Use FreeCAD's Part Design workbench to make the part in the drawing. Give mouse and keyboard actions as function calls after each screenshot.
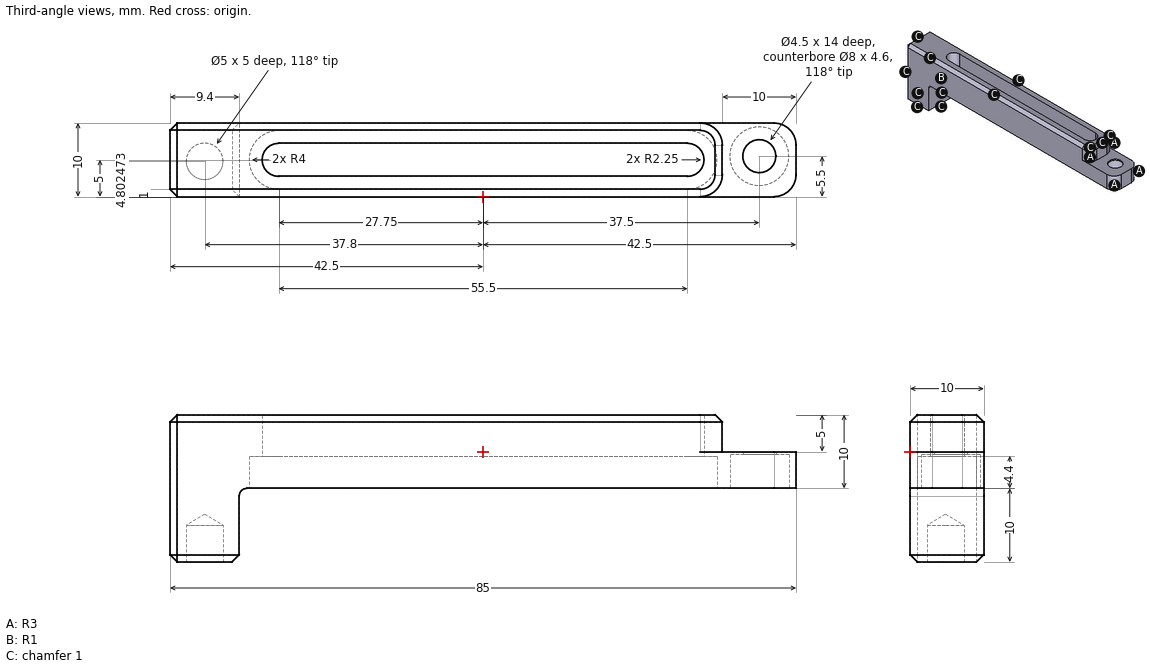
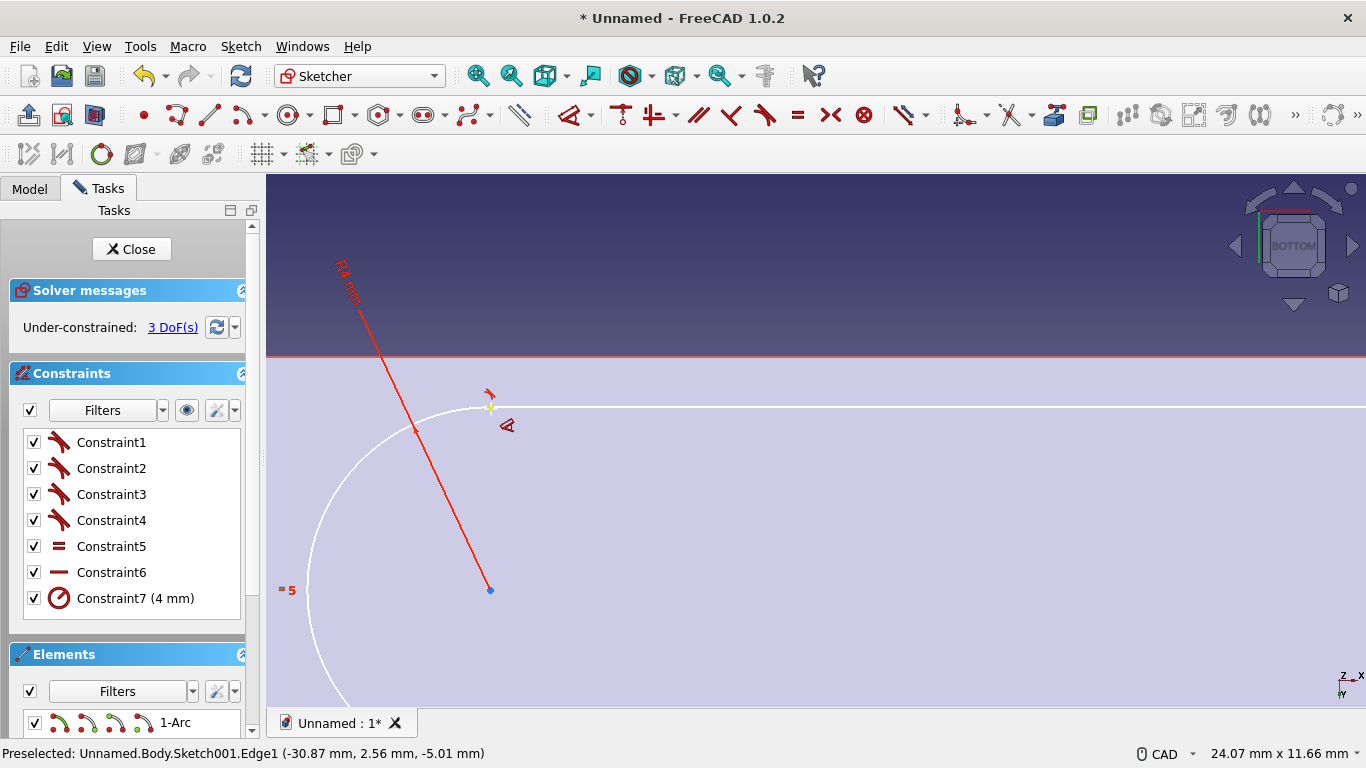
click(490, 407)
click(456, 382)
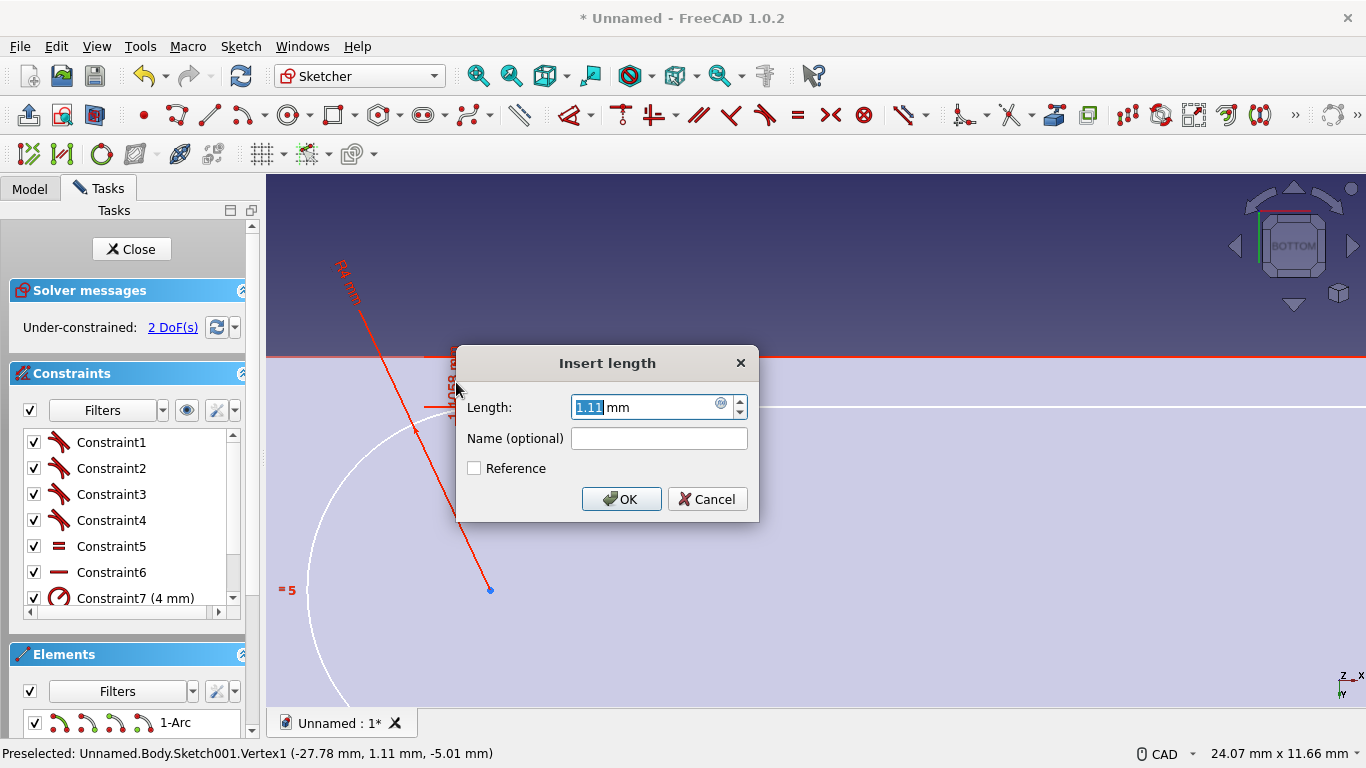
text(1)
key(Return)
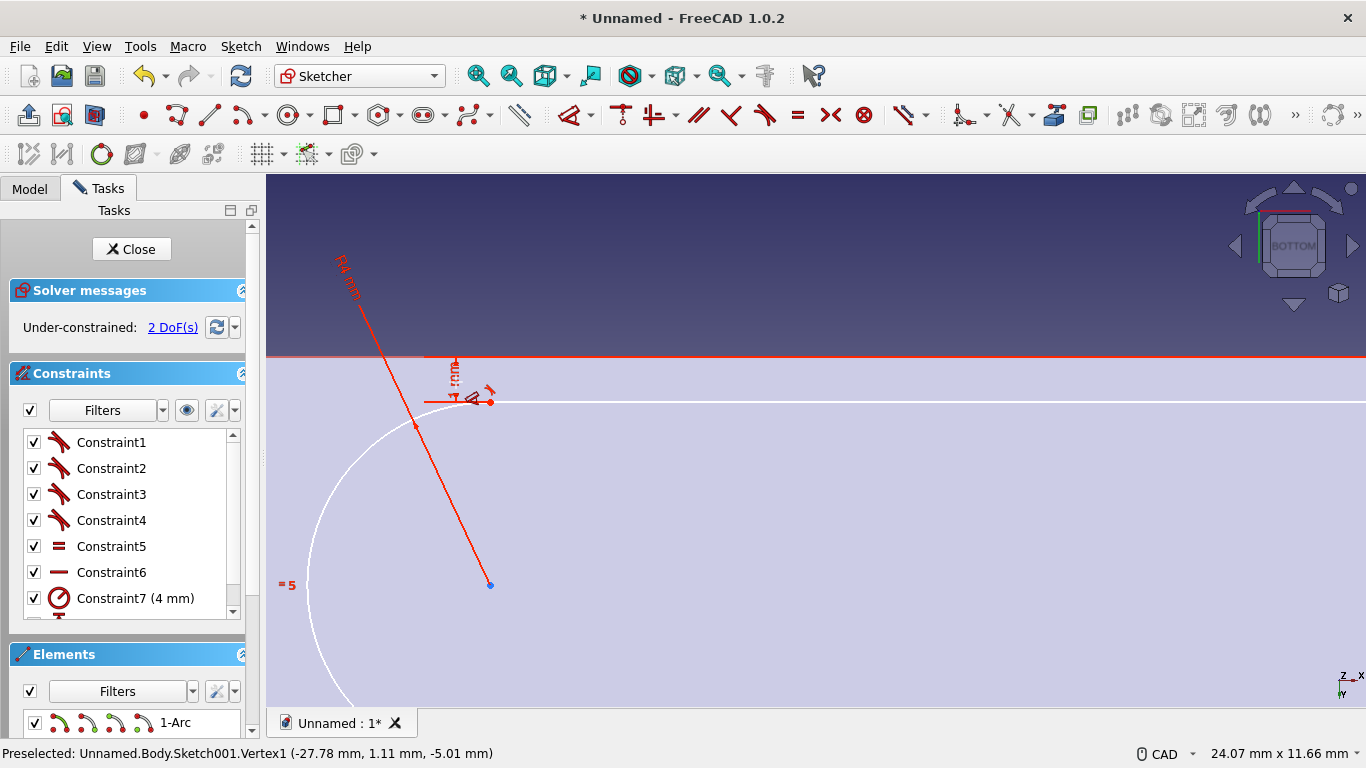
scroll(491, 410, down, 8)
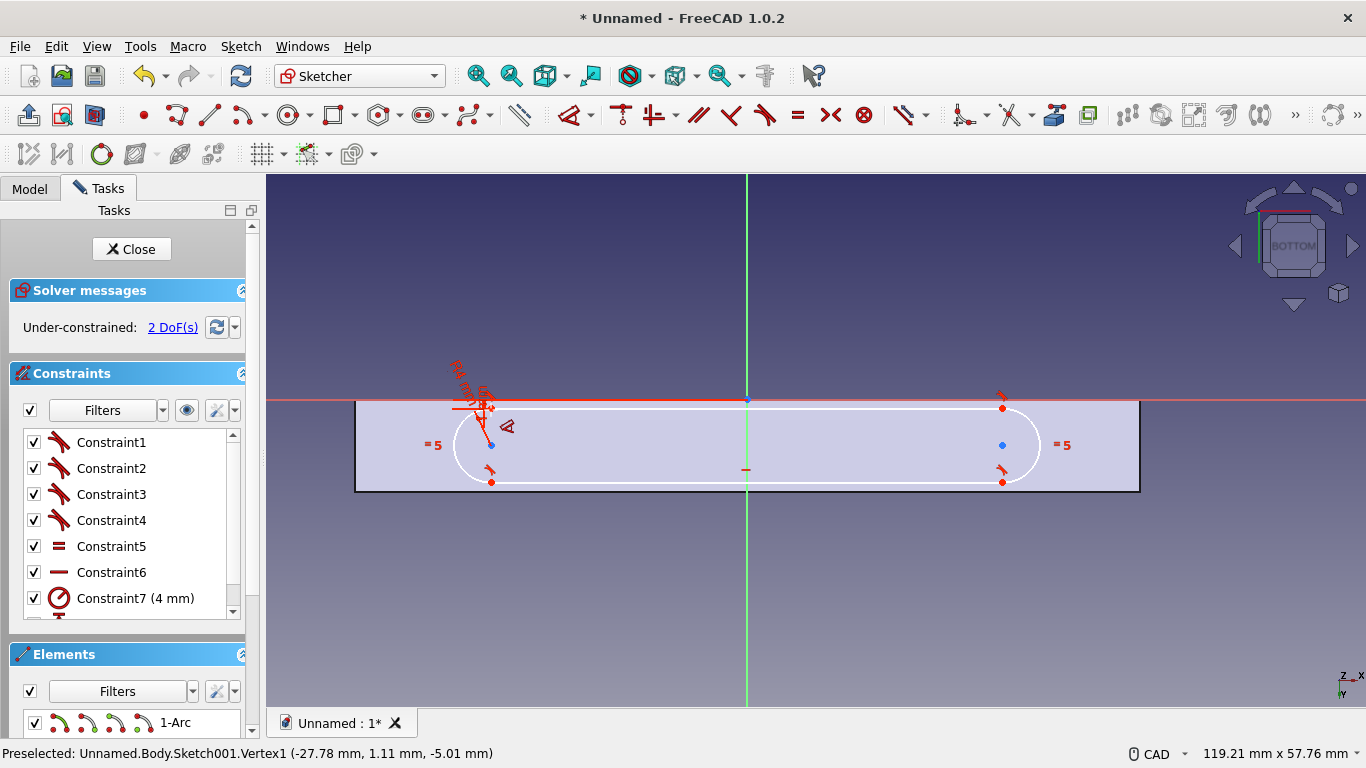
scroll(593, 409, up, 3)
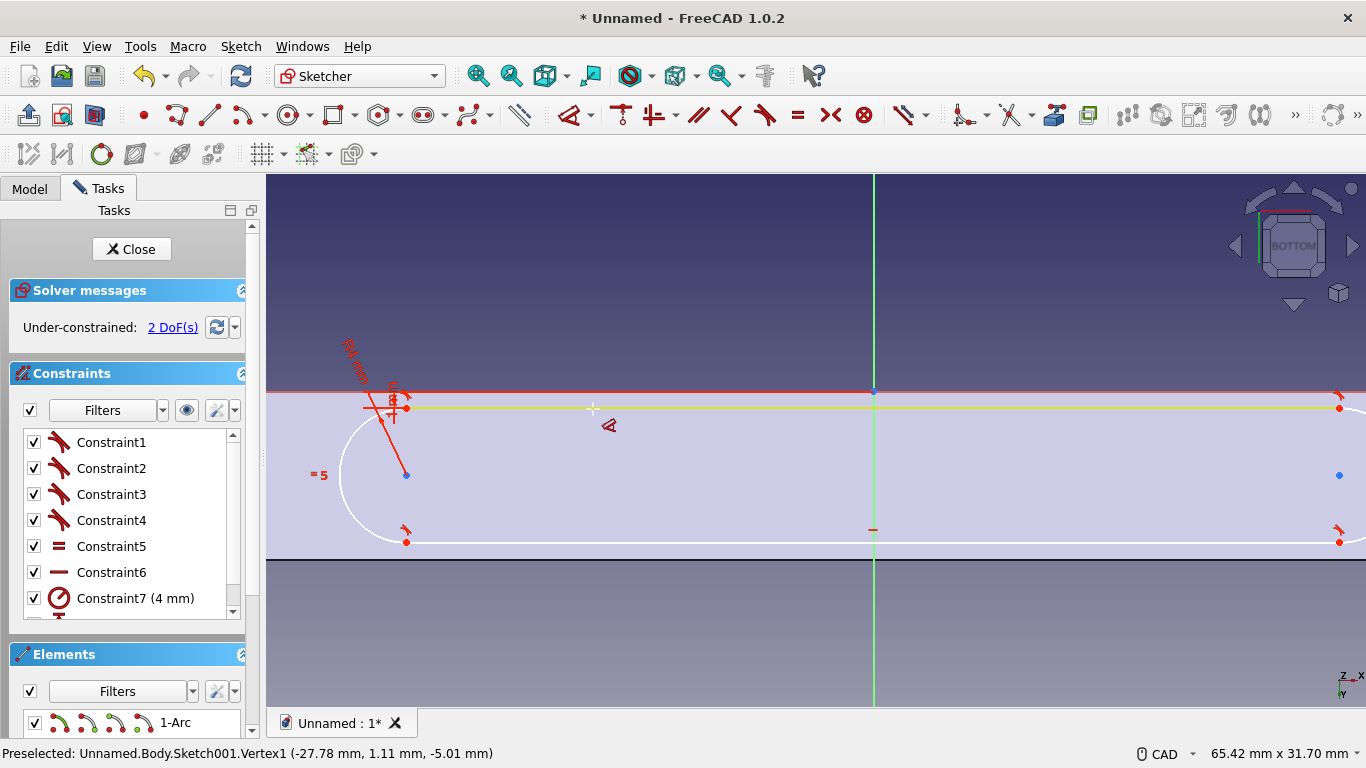
click(593, 408)
click(804, 374)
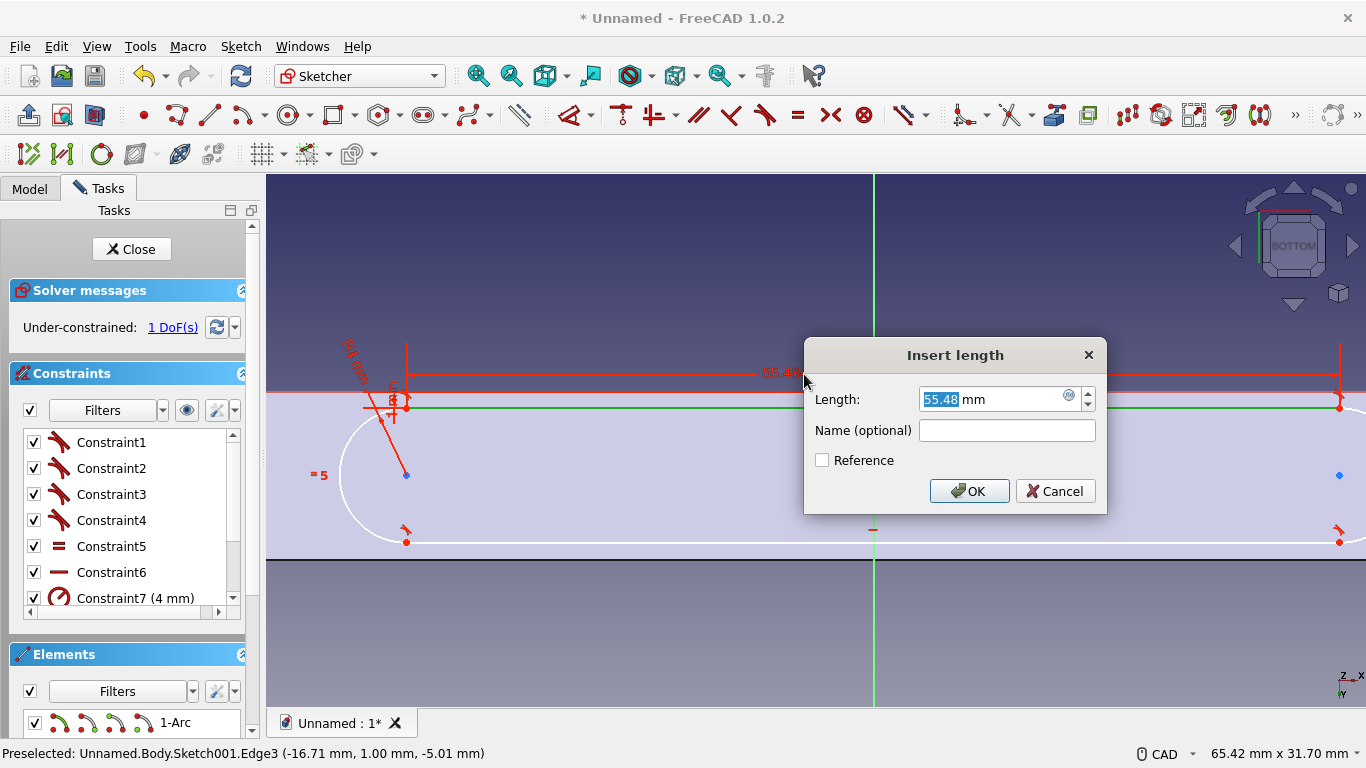
text(55.5)
key(Return)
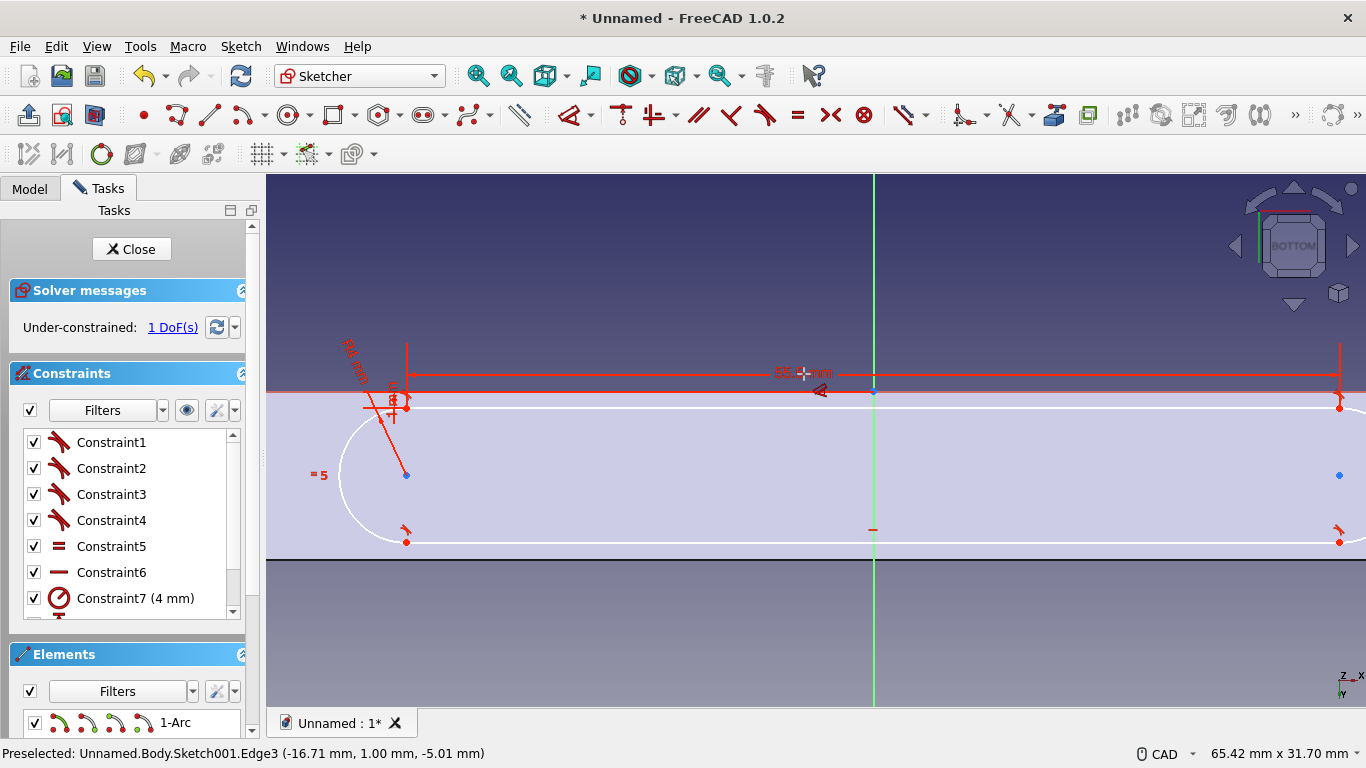
click(407, 408)
click(640, 358)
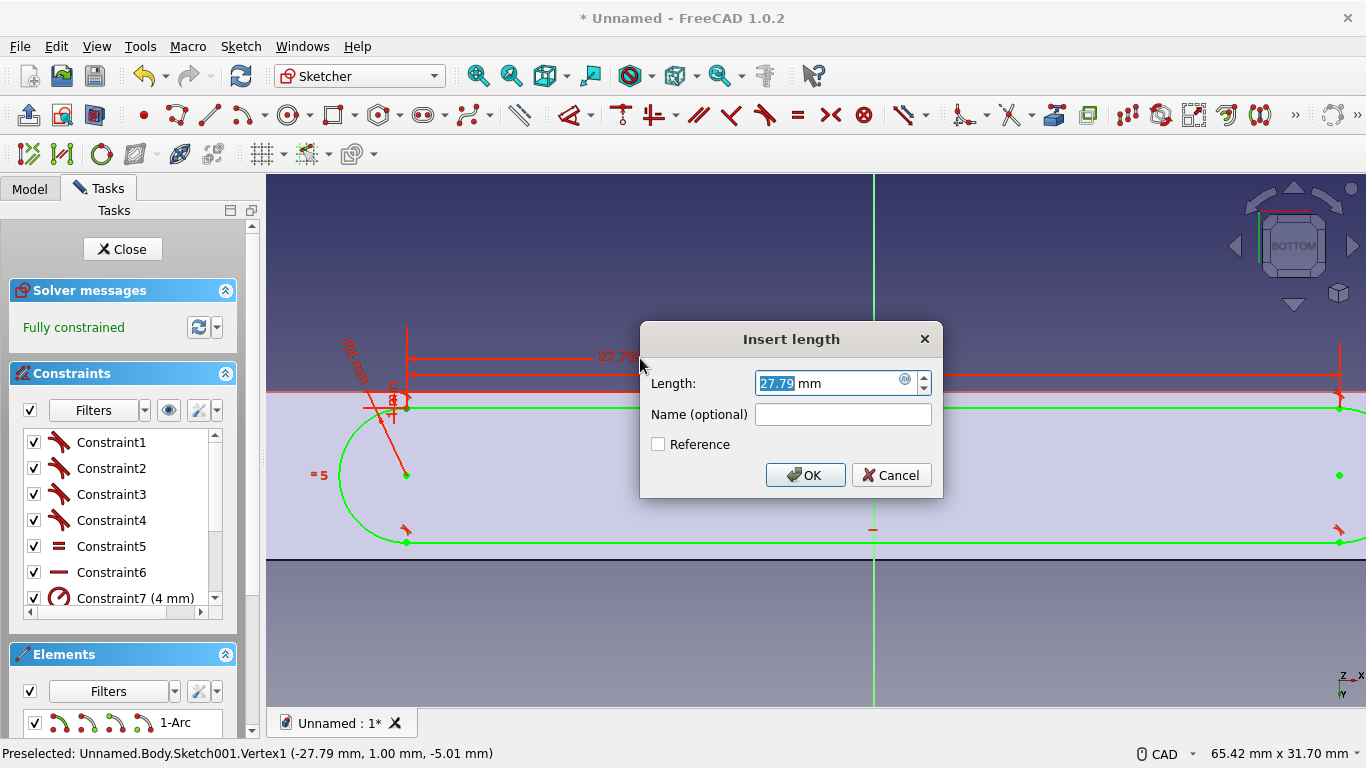
text(27.75)
key(Return)
key(Escape)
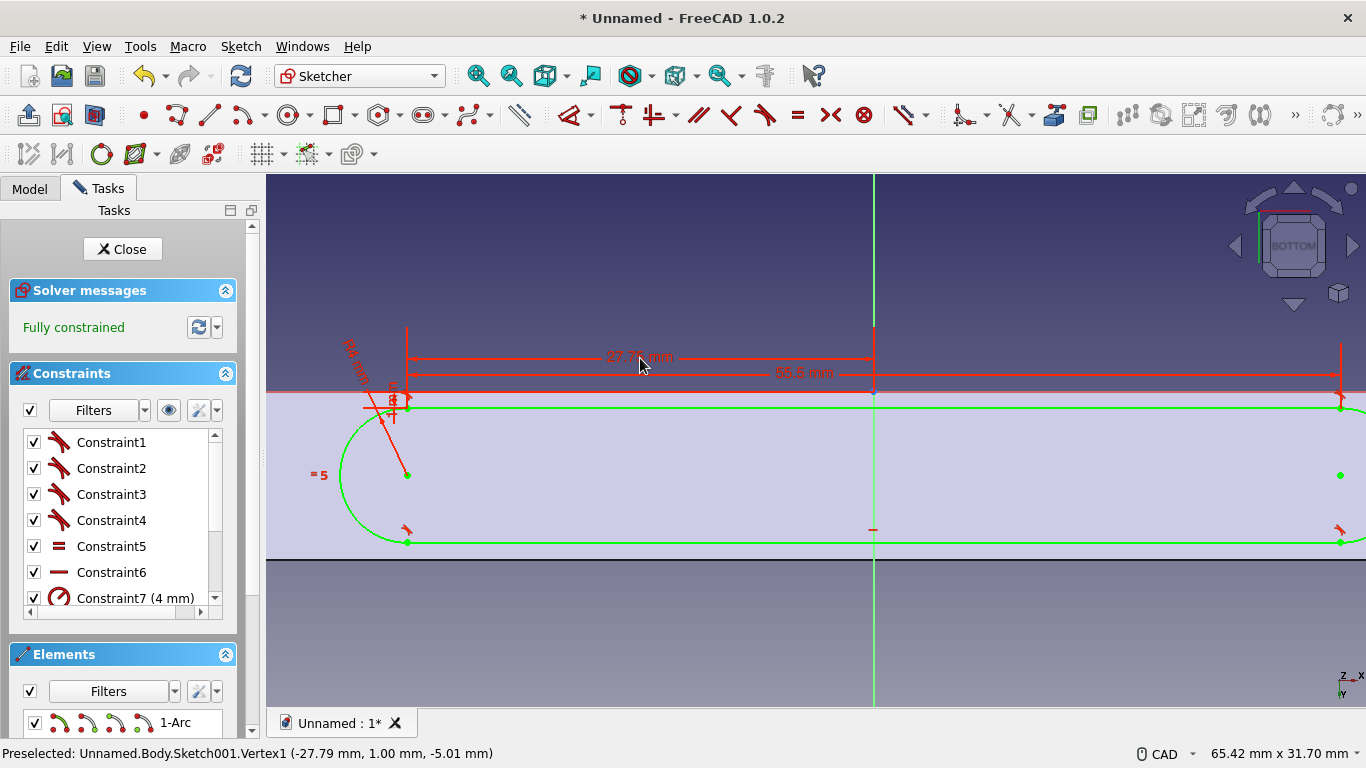
click(123, 249)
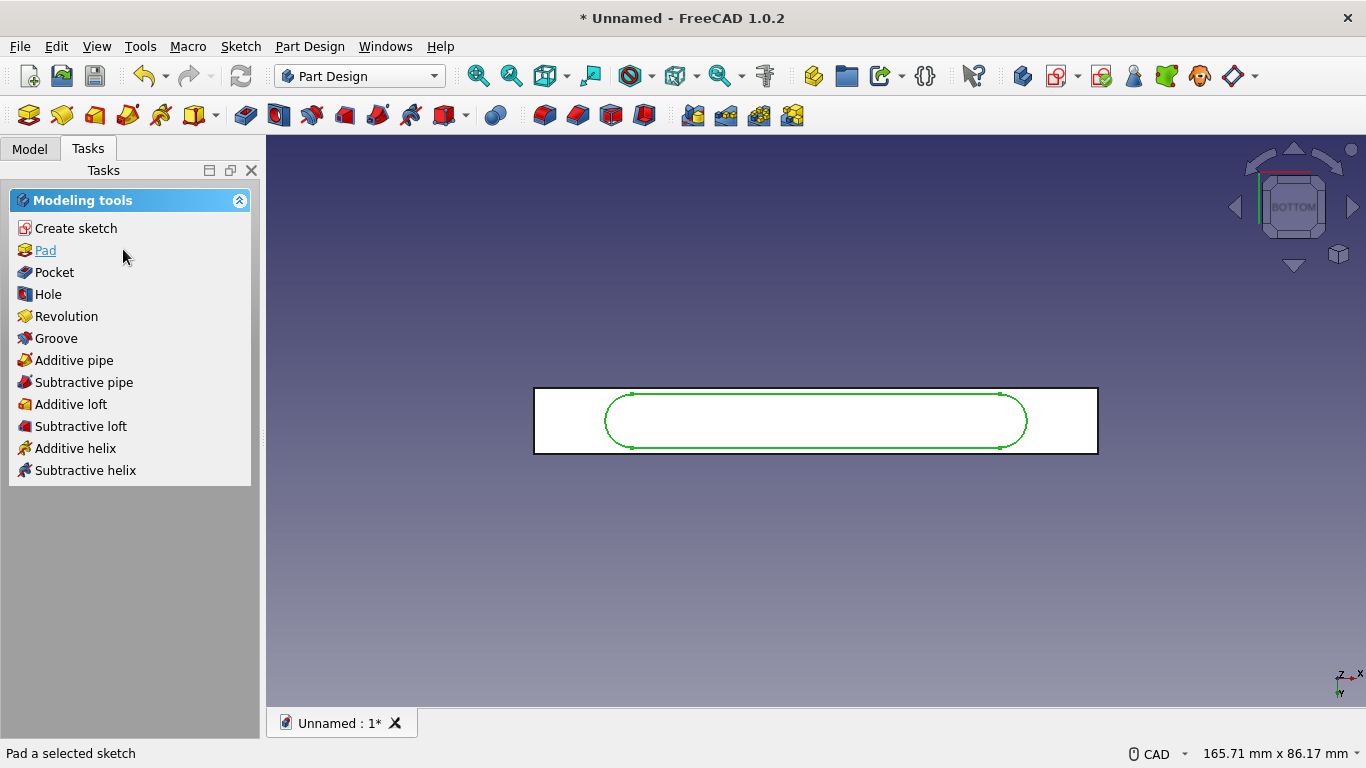
click(246, 116)